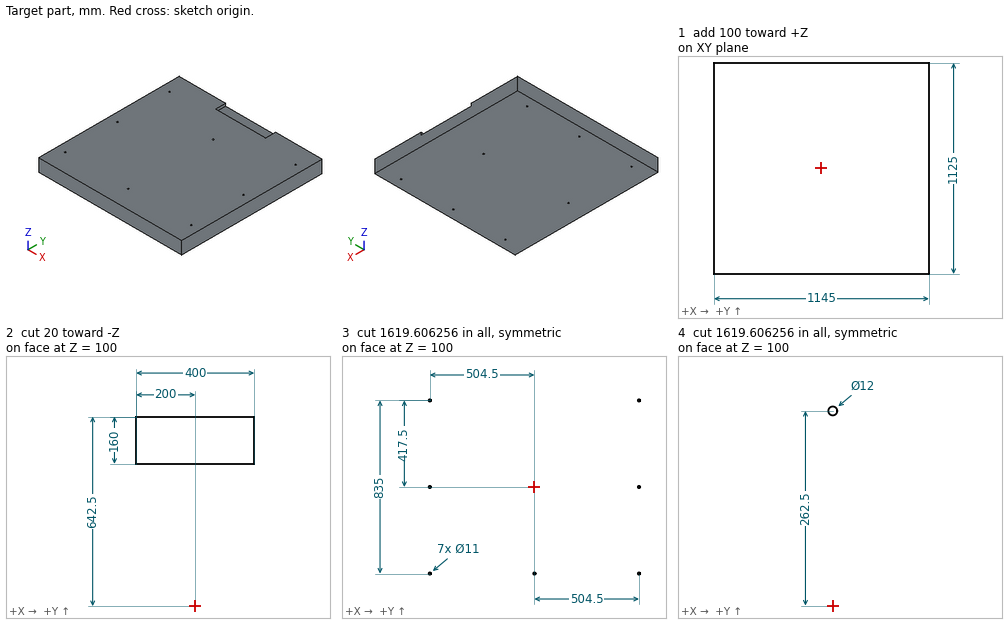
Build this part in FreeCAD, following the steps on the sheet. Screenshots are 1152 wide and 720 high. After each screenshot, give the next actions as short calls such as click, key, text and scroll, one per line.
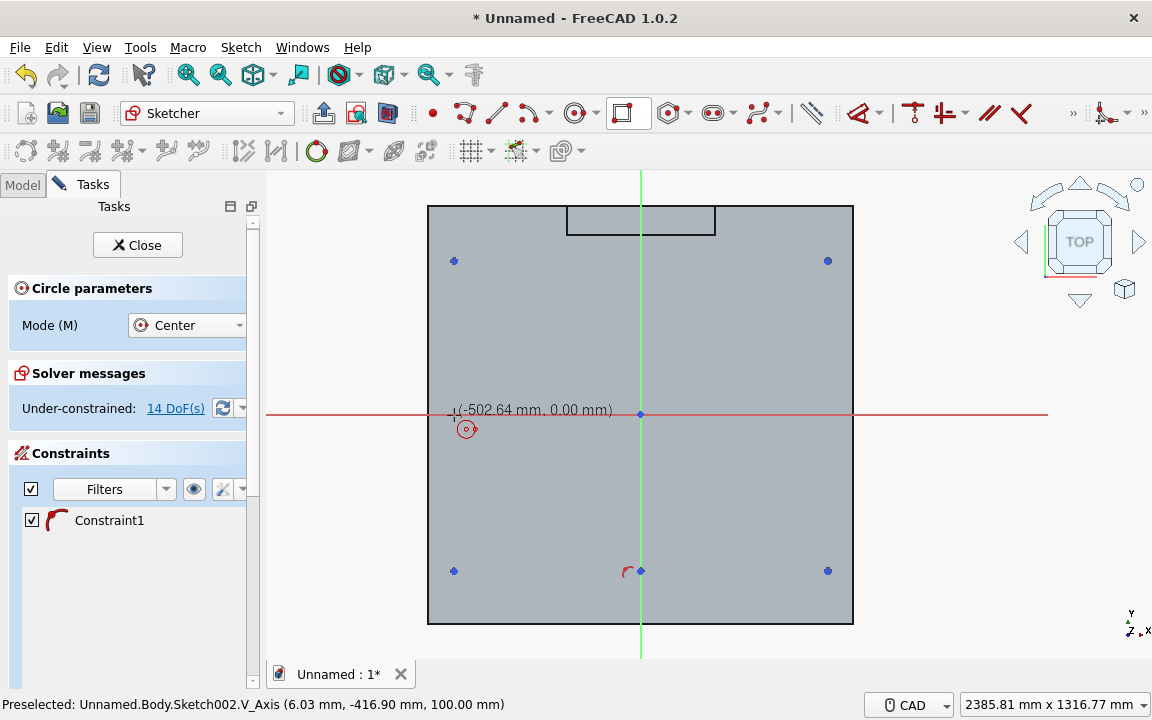
click(454, 415)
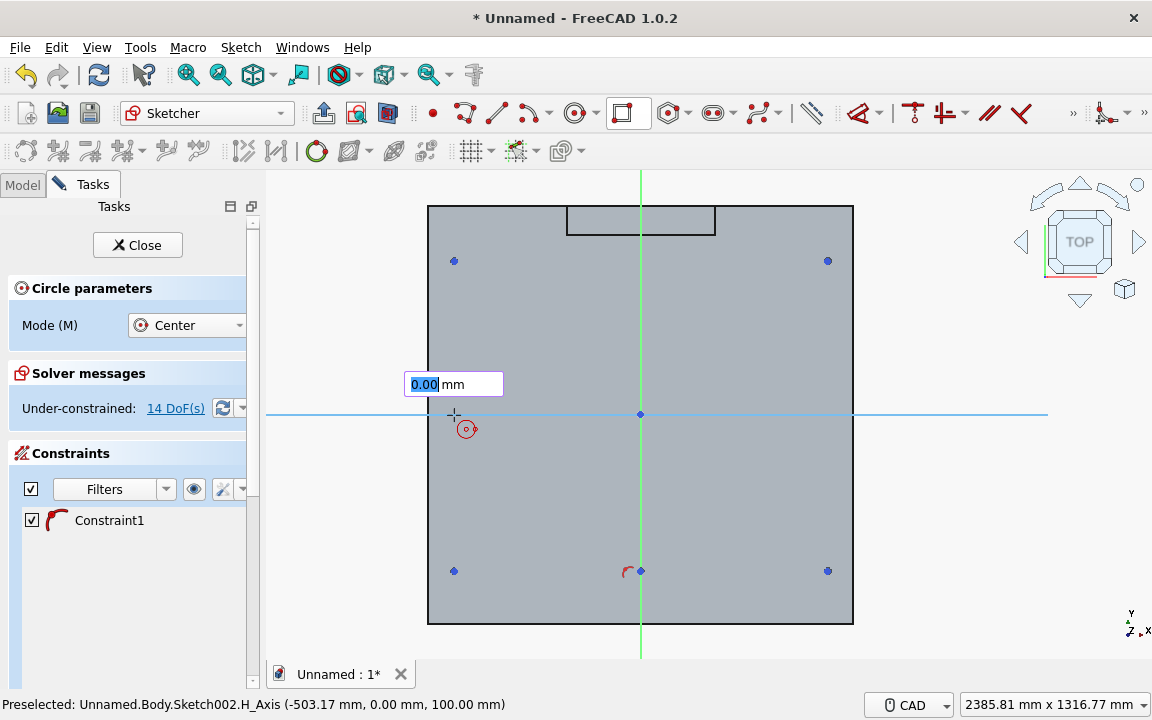
scroll(454, 413, up, 11)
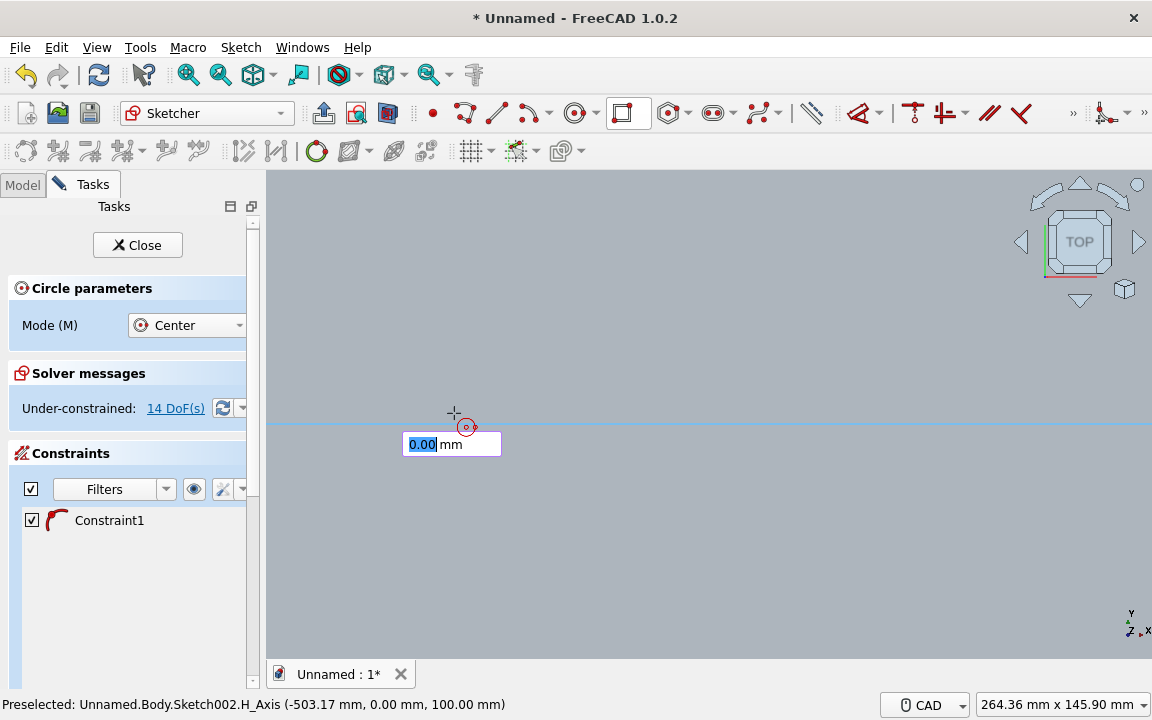
click(454, 406)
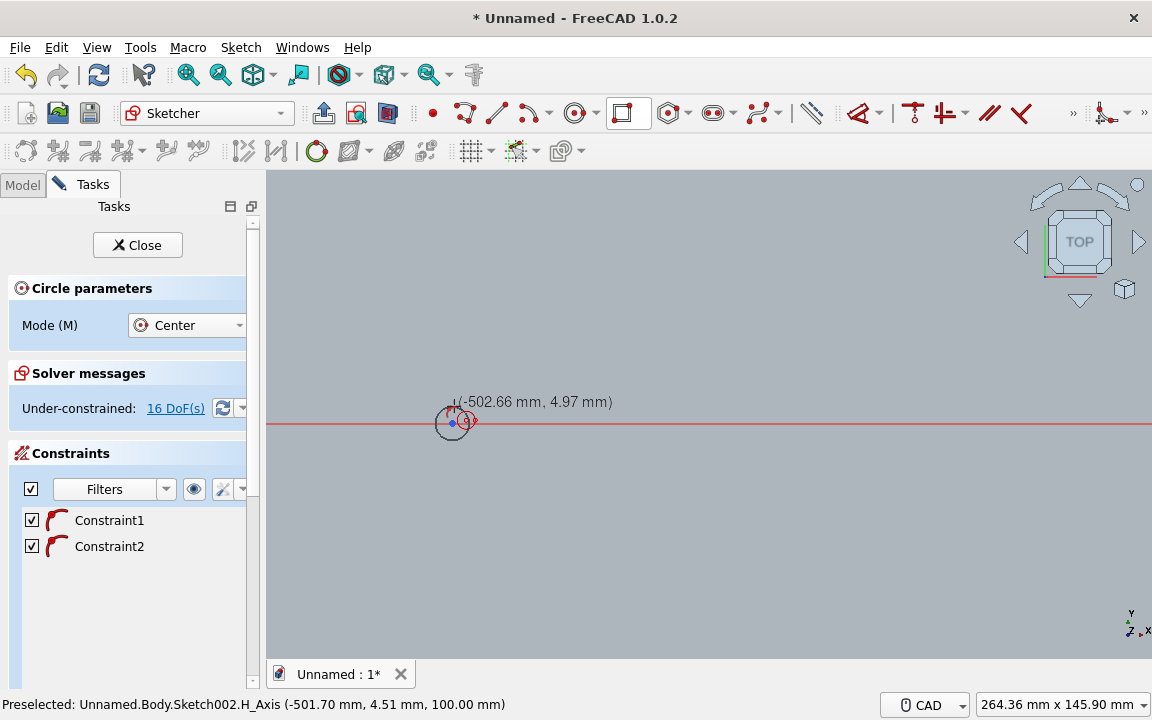
scroll(454, 413, down, 11)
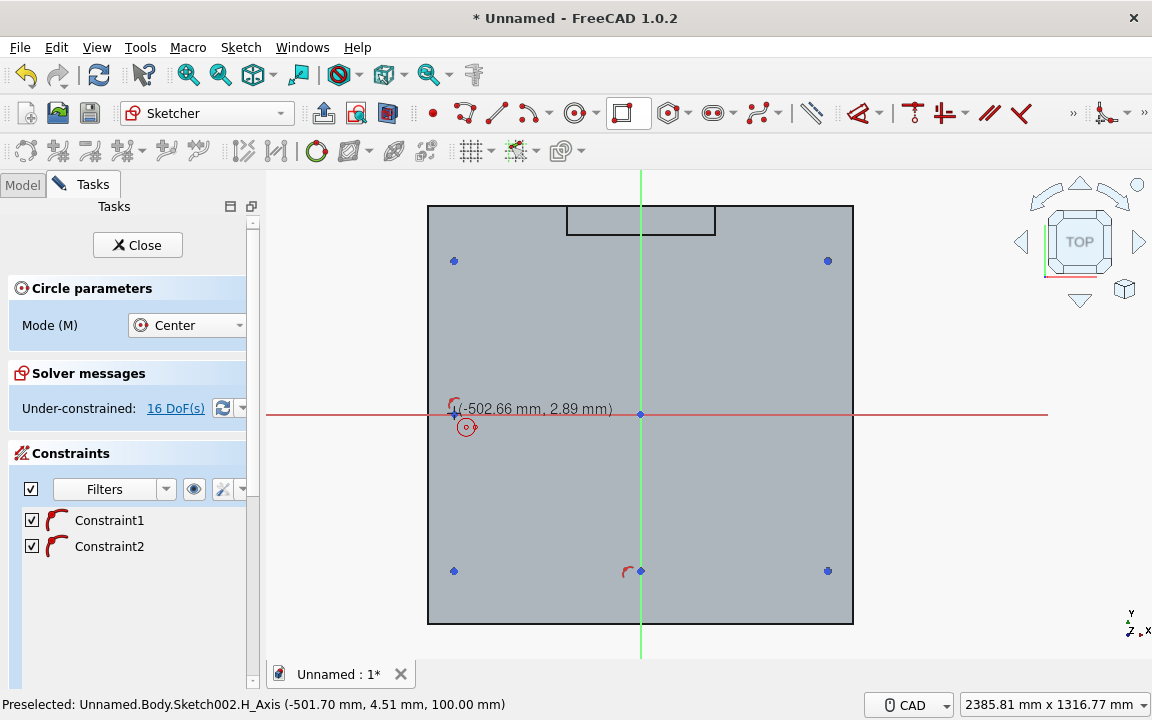
scroll(828, 415, up, 13)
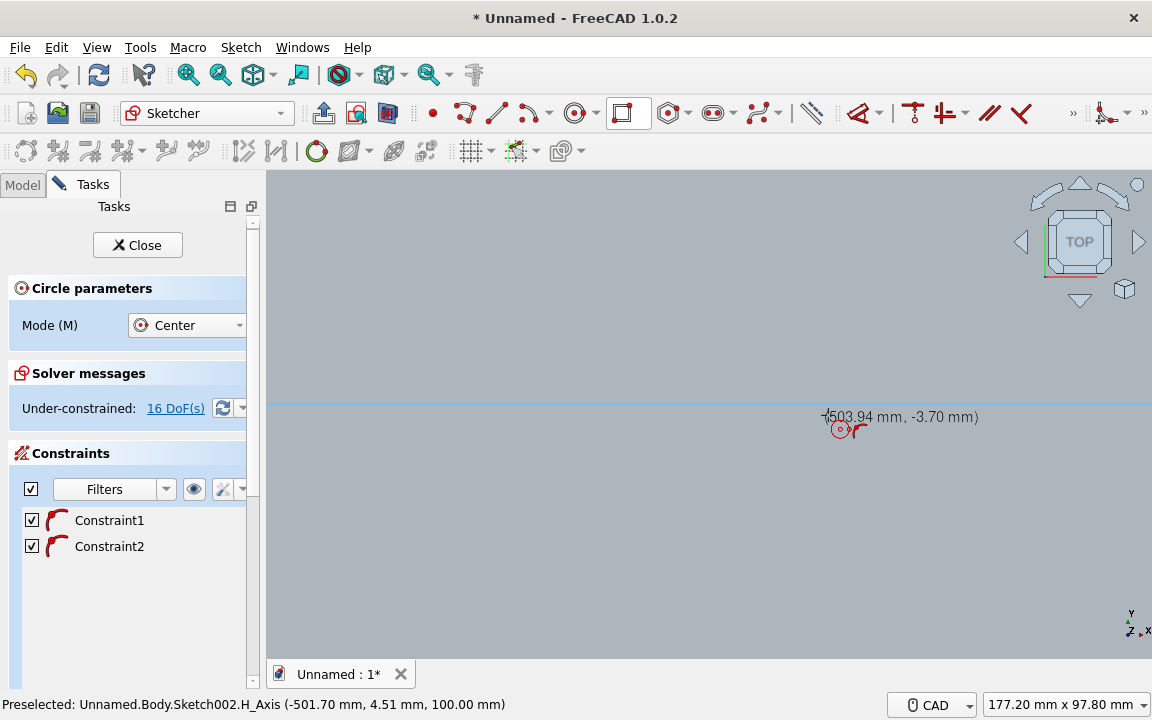
scroll(828, 415, down, 13)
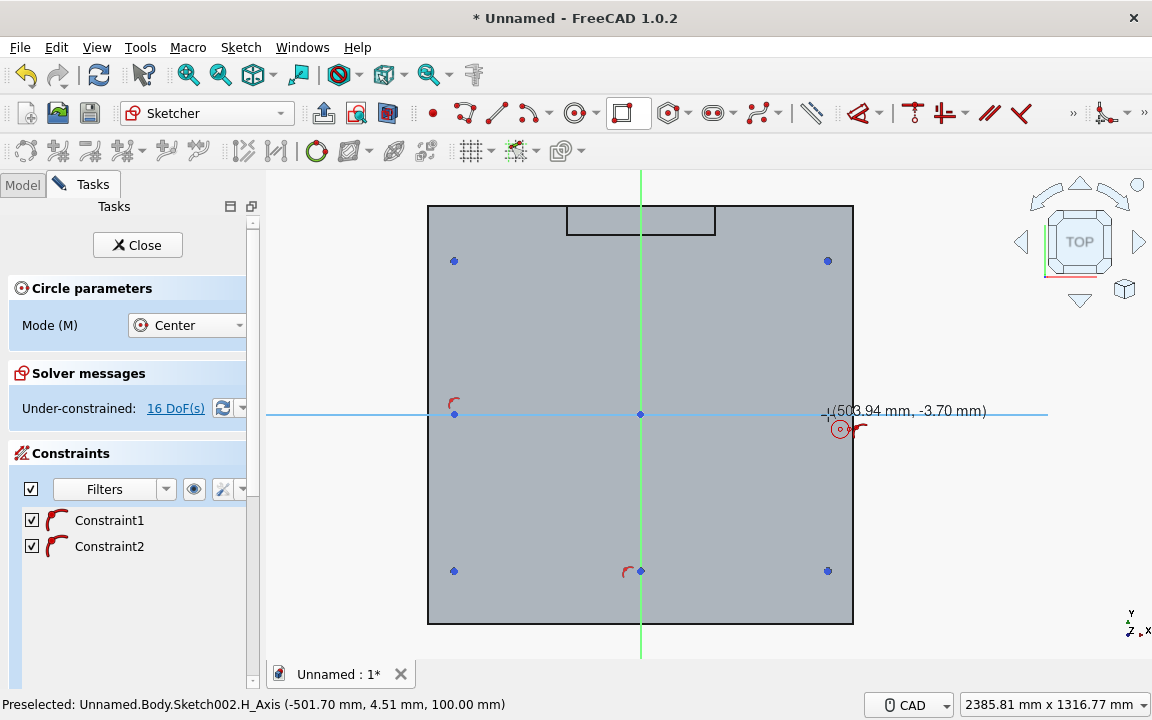
click(828, 415)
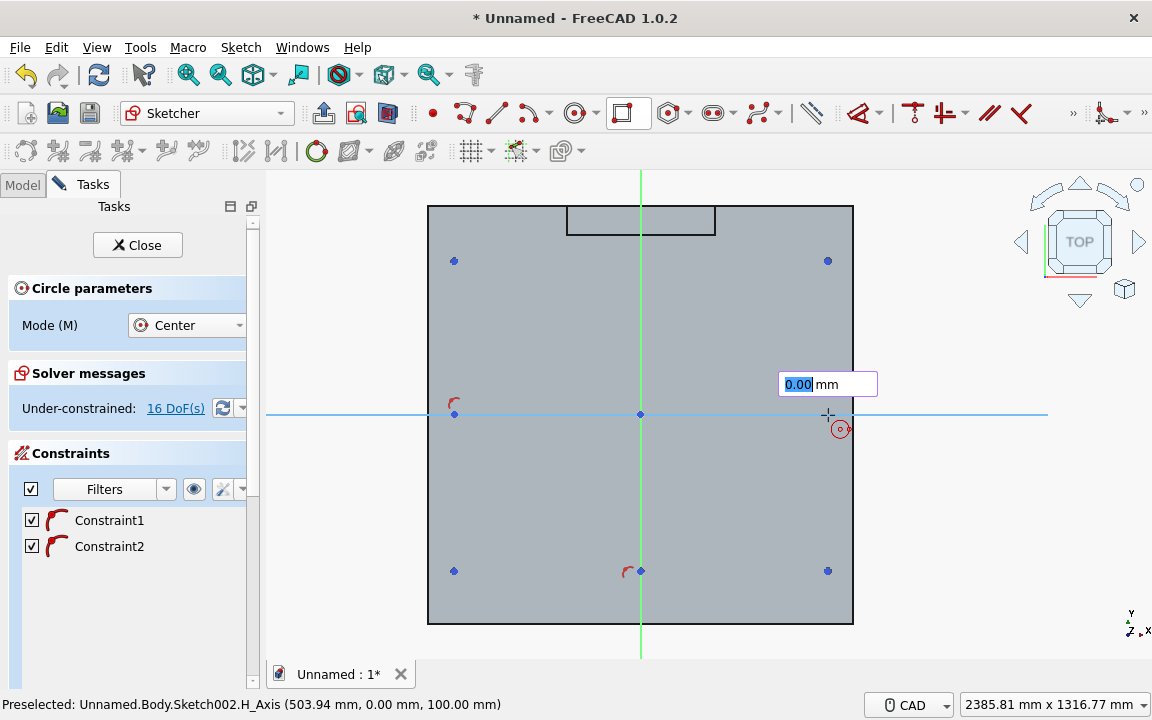
scroll(829, 413, up, 11)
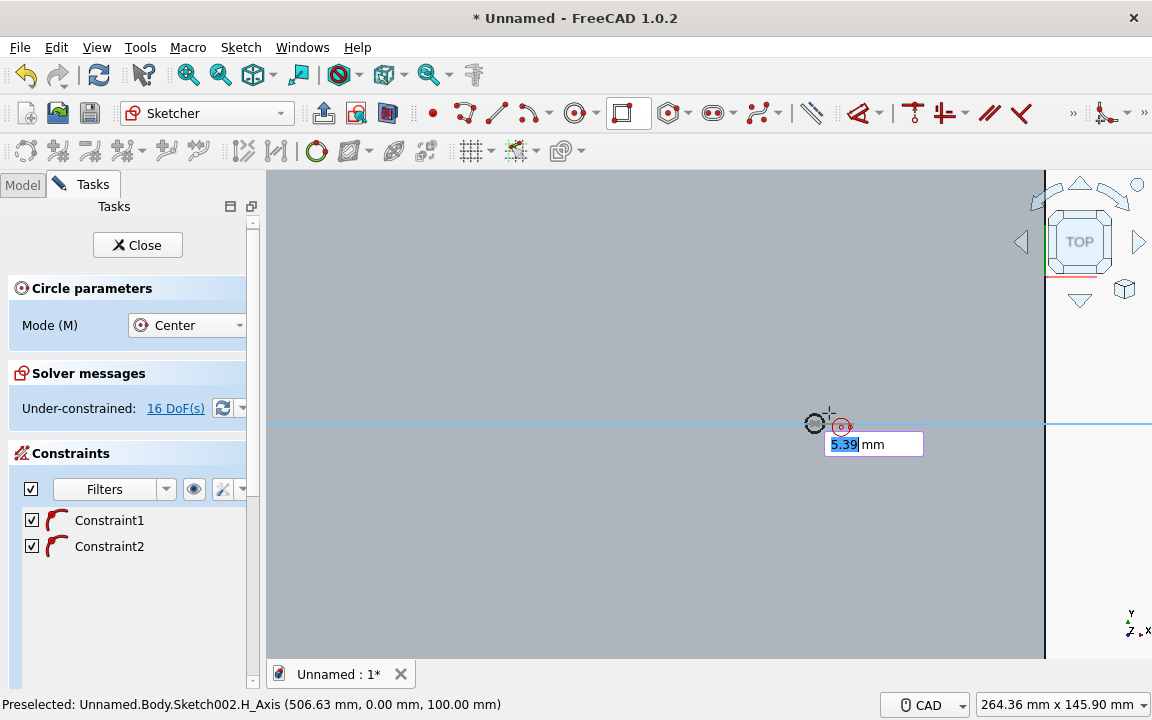
click(823, 406)
key(Escape)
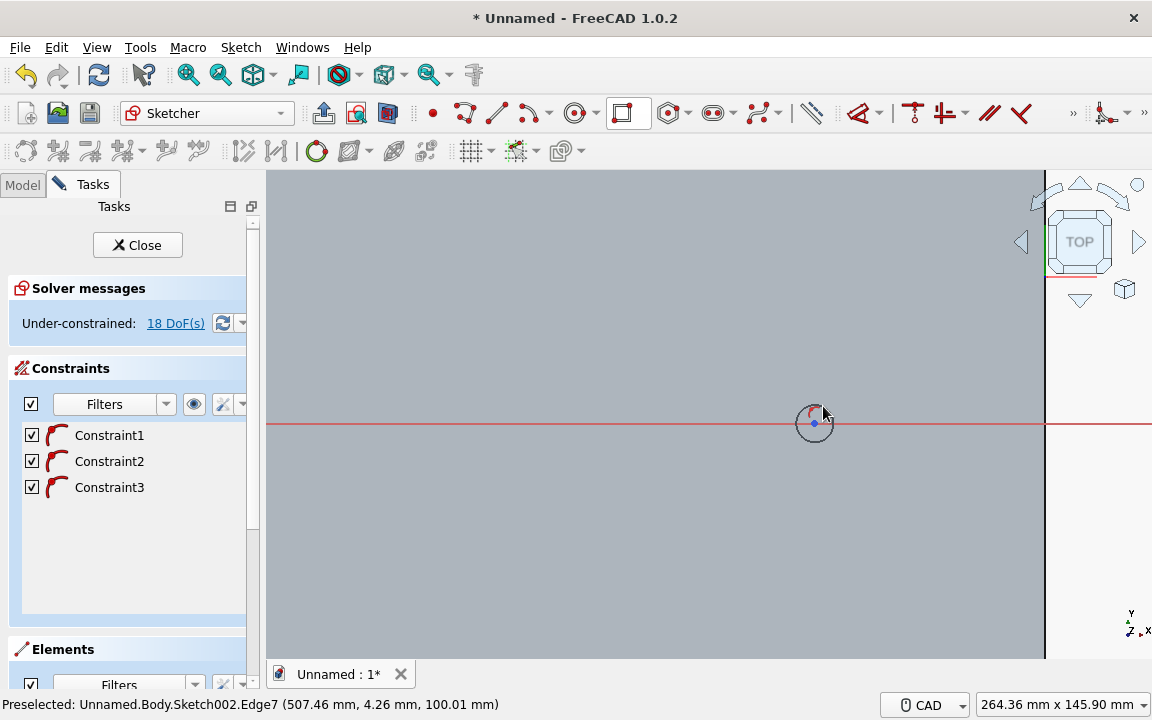
scroll(829, 413, down, 11)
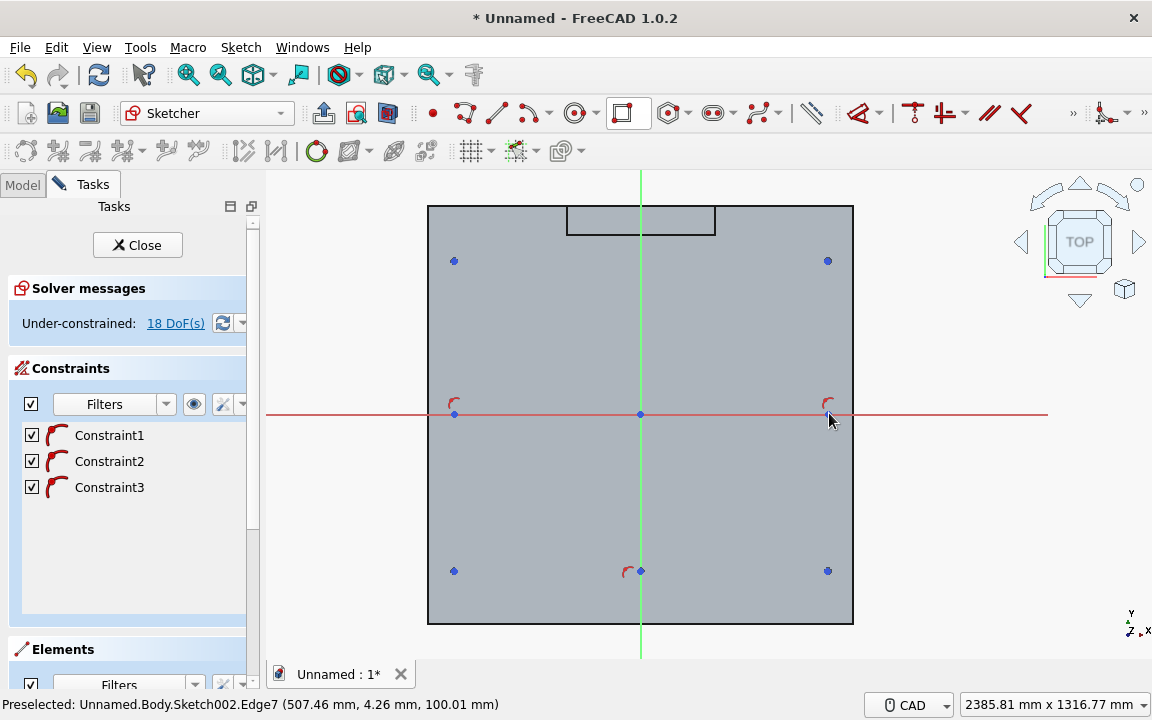
scroll(456, 259, up, 8)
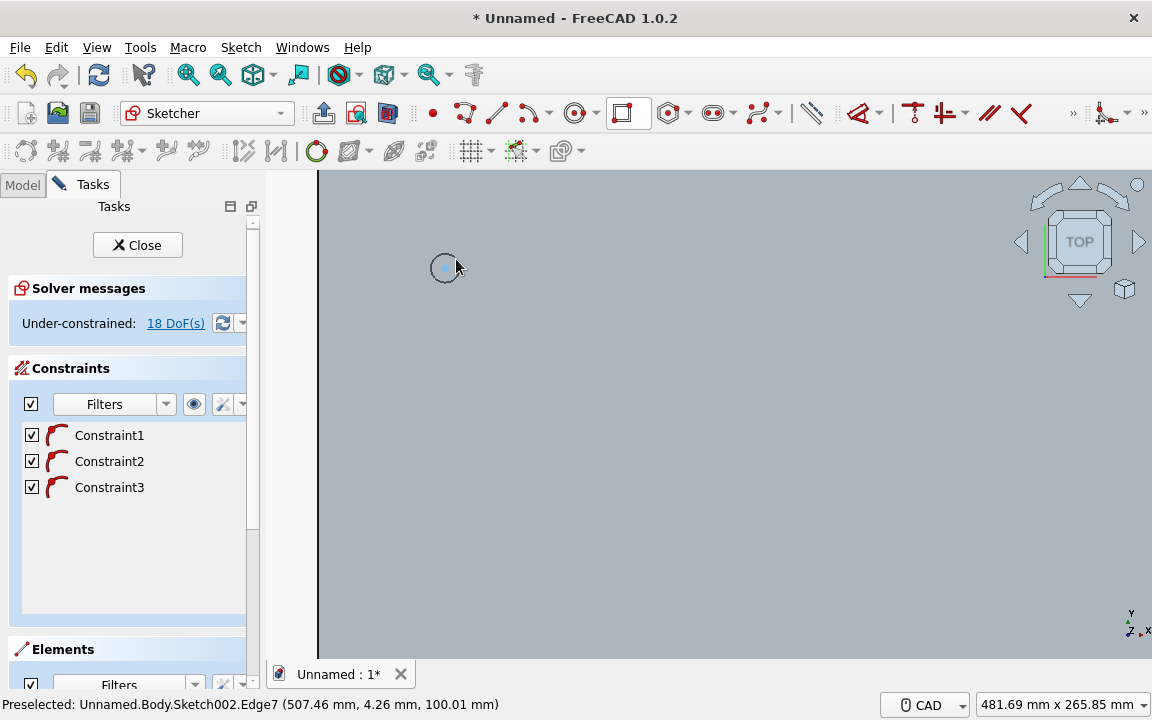
click(455, 258)